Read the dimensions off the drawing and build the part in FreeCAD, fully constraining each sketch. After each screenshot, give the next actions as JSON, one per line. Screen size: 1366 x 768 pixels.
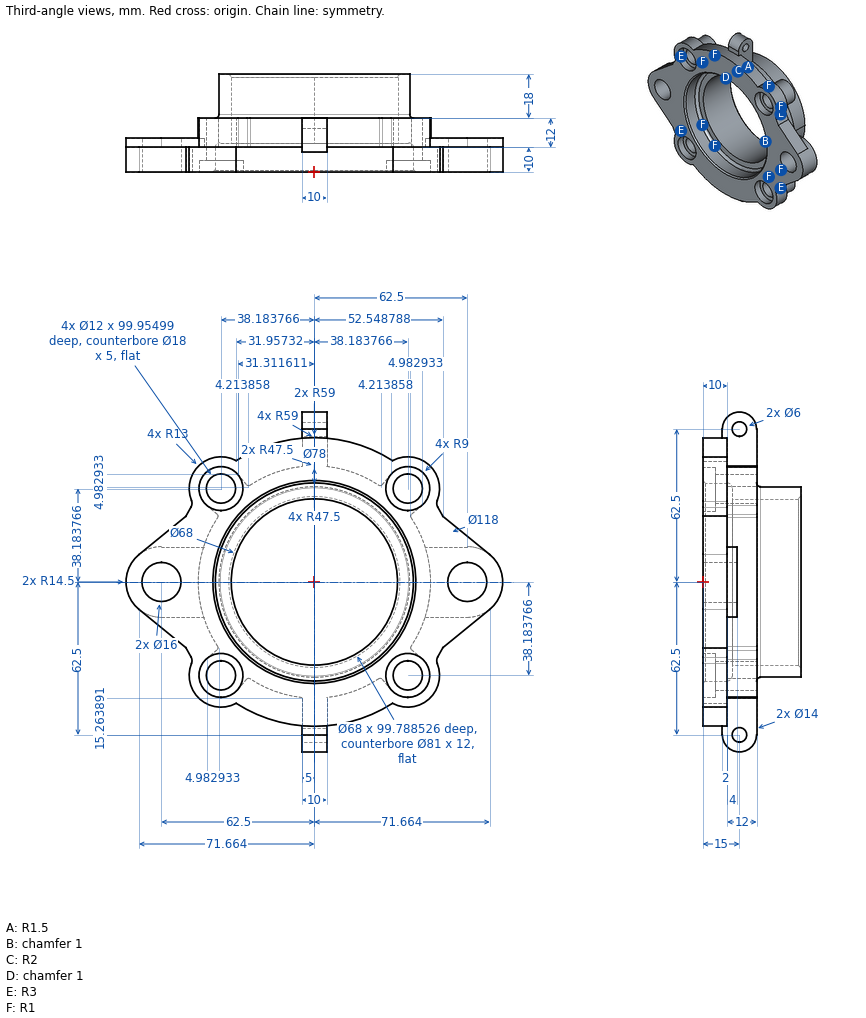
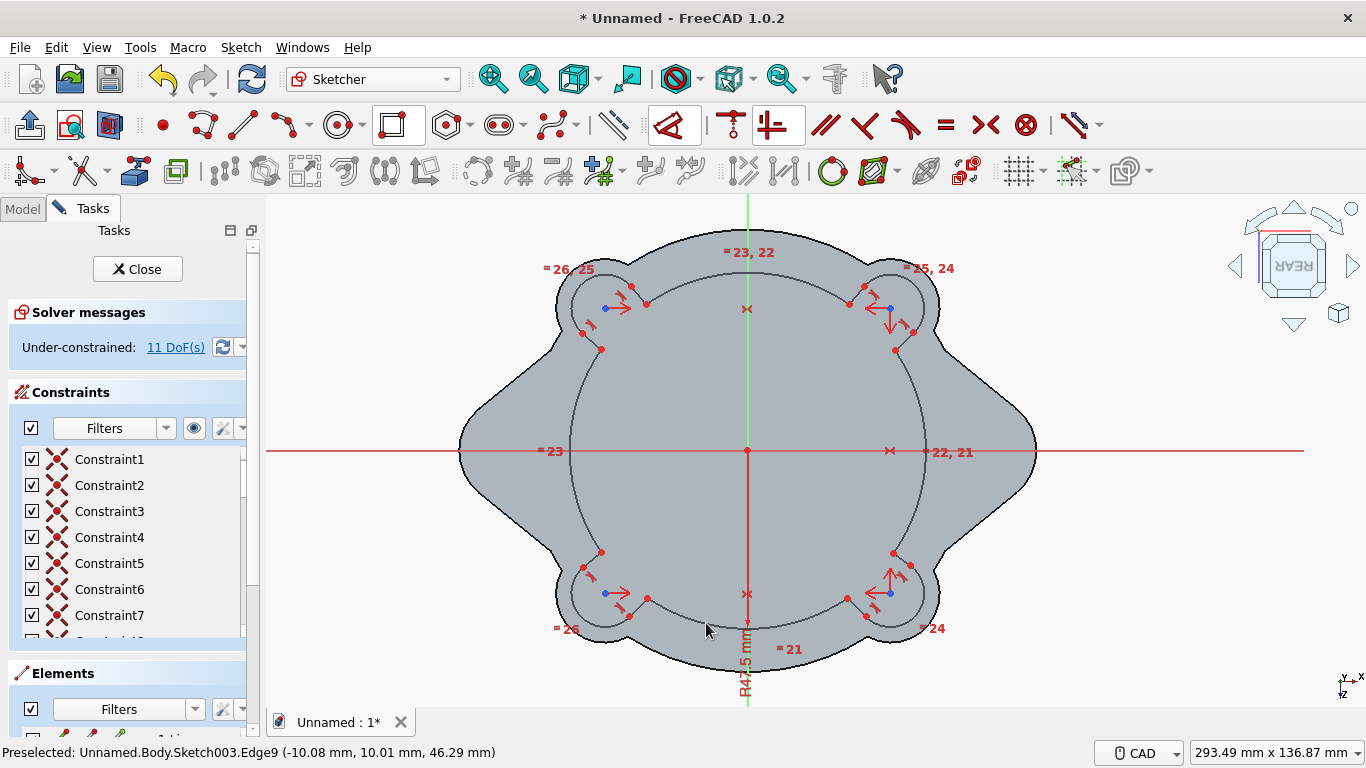
{"action": "left_click", "coordinate": [897, 626]}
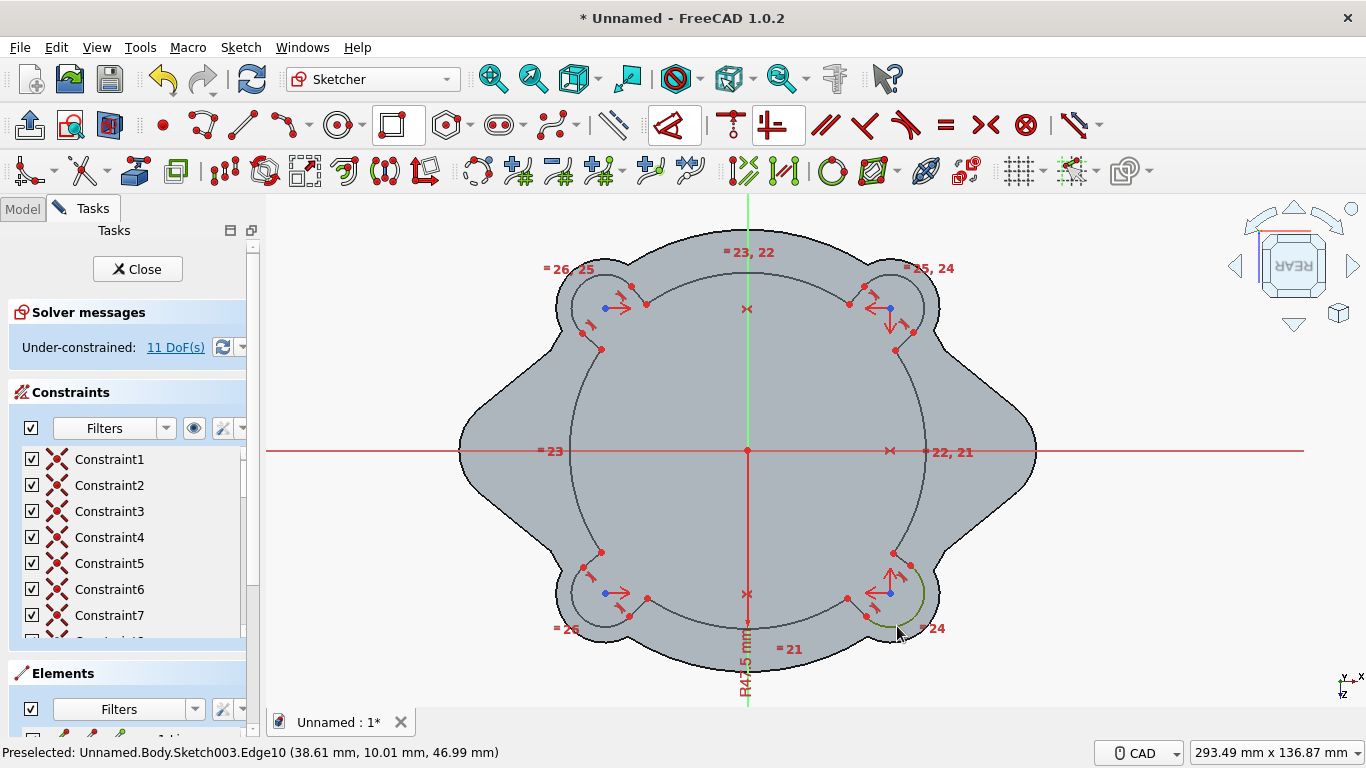
{"action": "key", "text": "k r"}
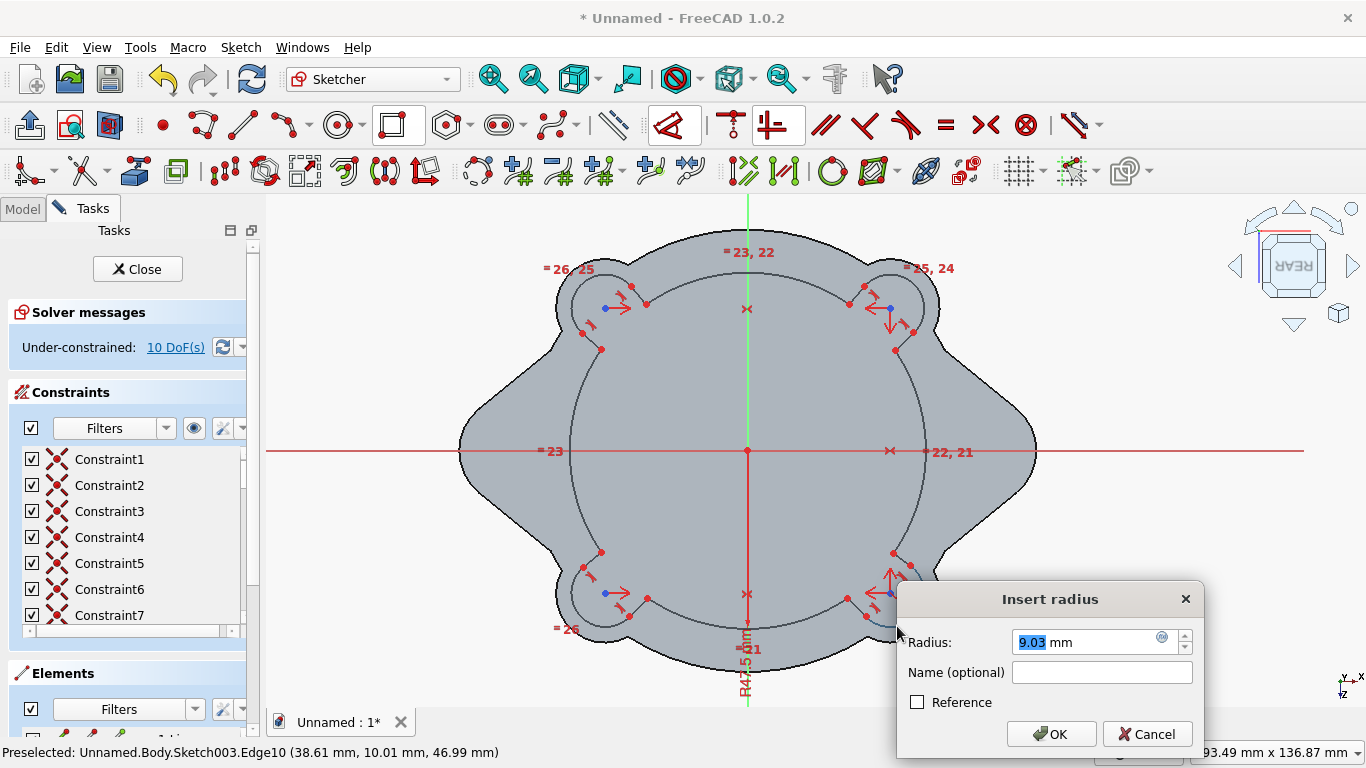
{"action": "type", "text": "9"}
{"action": "key", "text": "Return"}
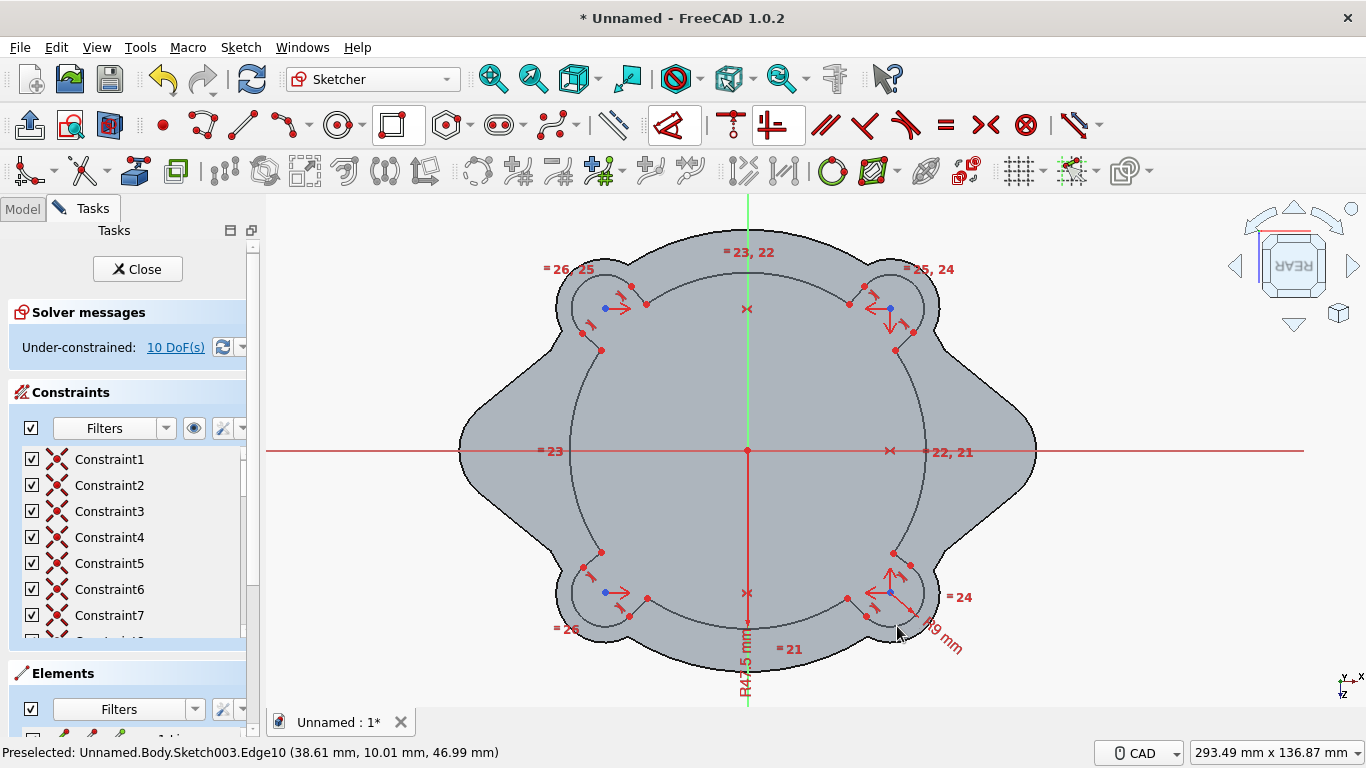
{"action": "scroll", "coordinate": [637, 609], "scroll_direction": "up", "scroll_amount": 5}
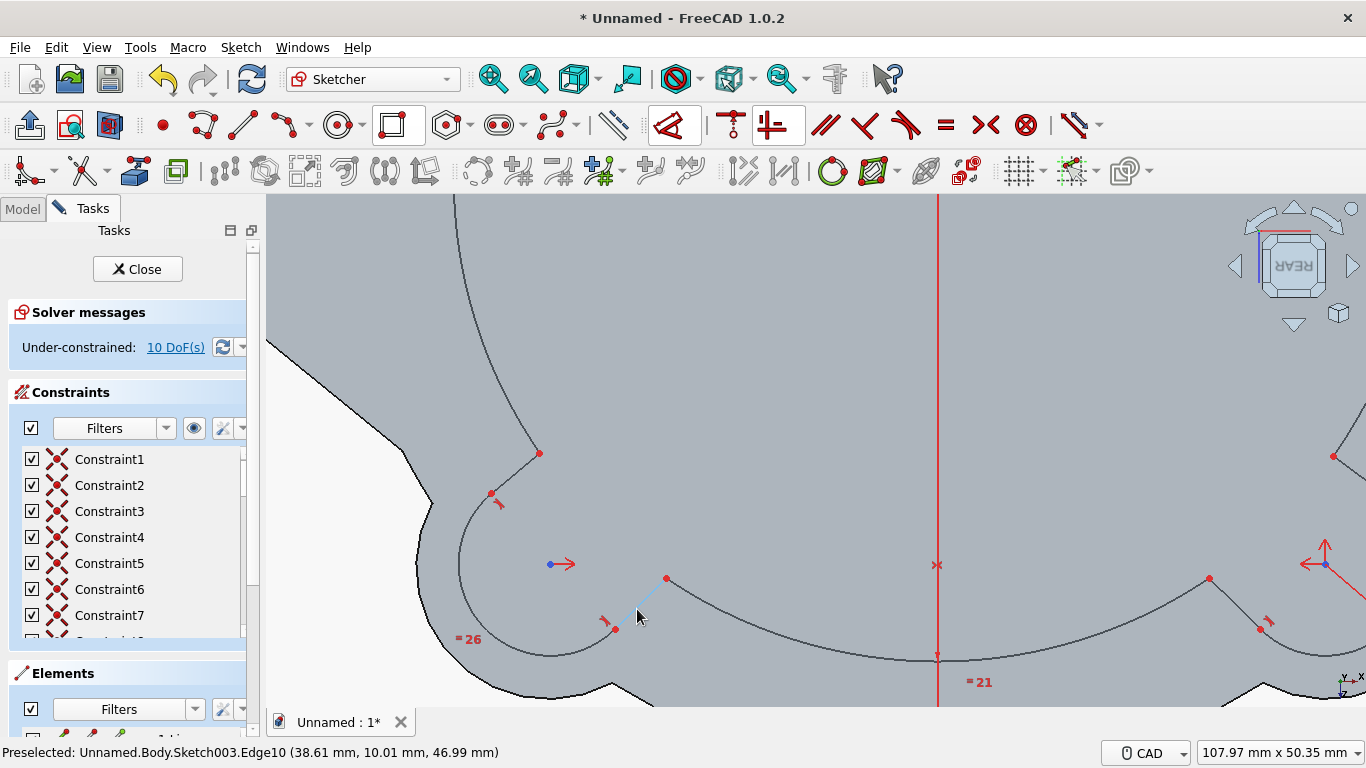
{"action": "left_click", "coordinate": [635, 609]}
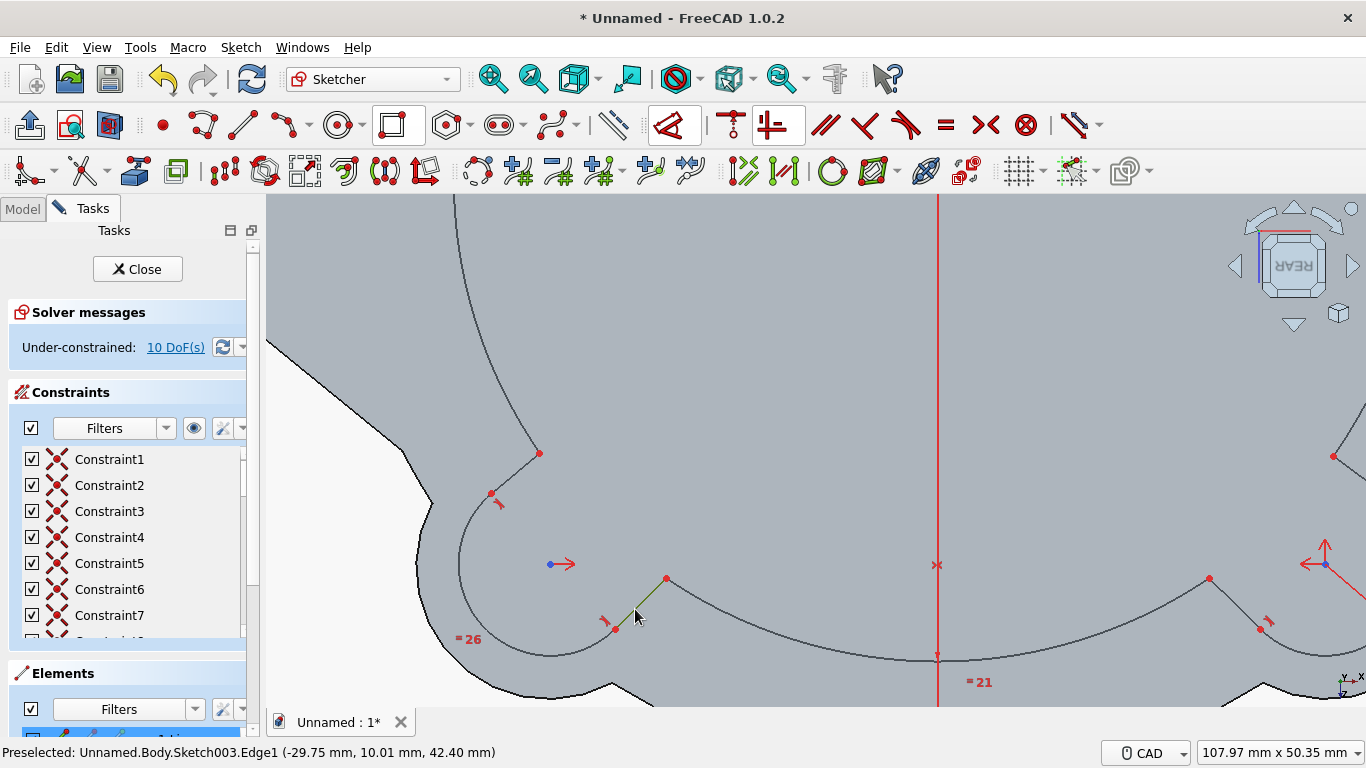
{"action": "left_click", "coordinate": [696, 126]}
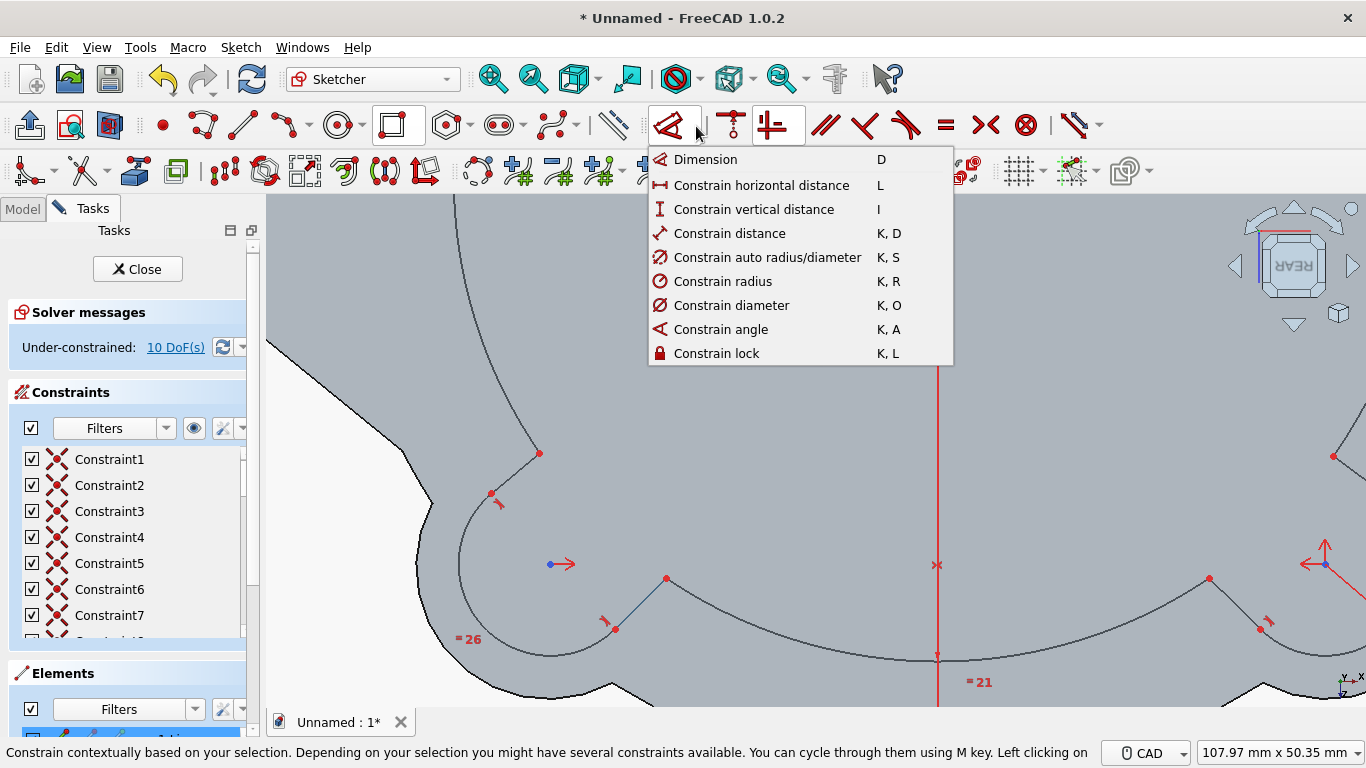
{"action": "left_click", "coordinate": [801, 185]}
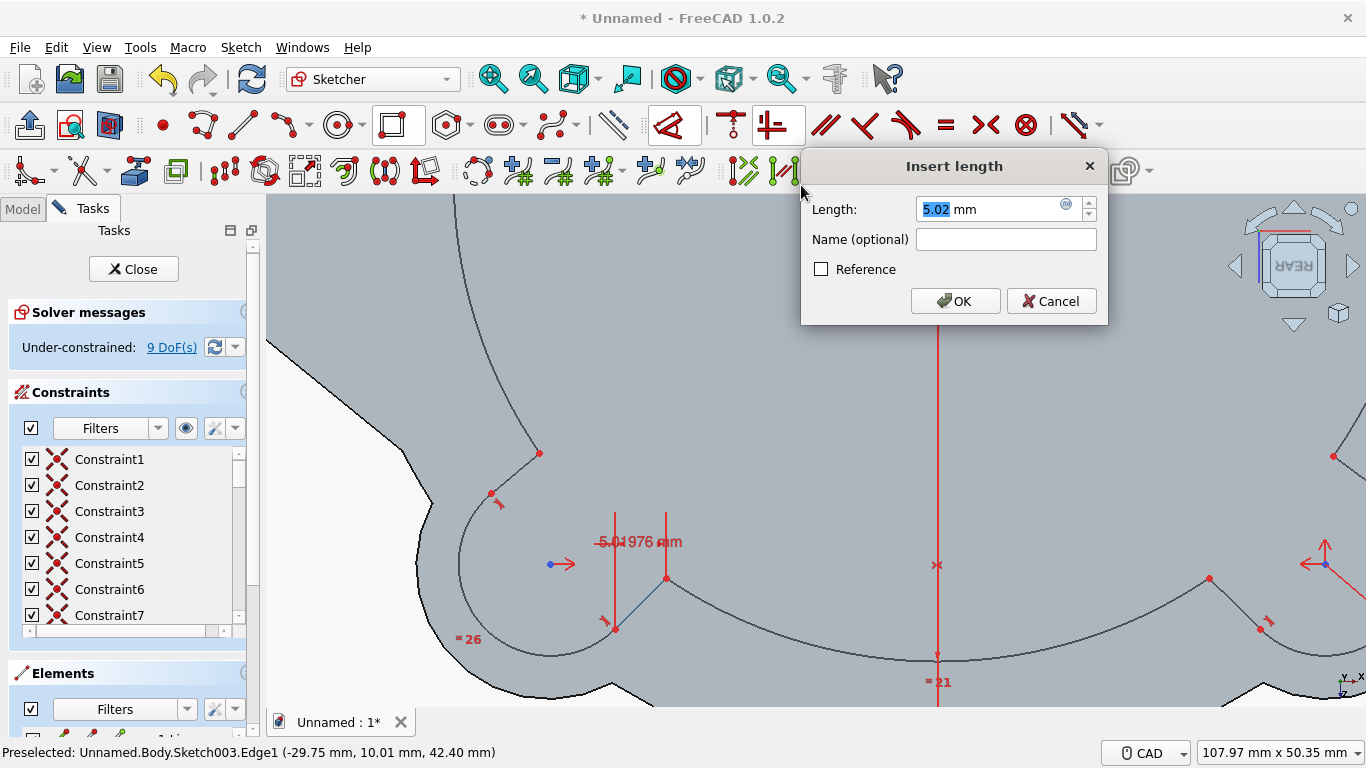
{"action": "type", "text": "4.213858"}
{"action": "key", "text": "Return"}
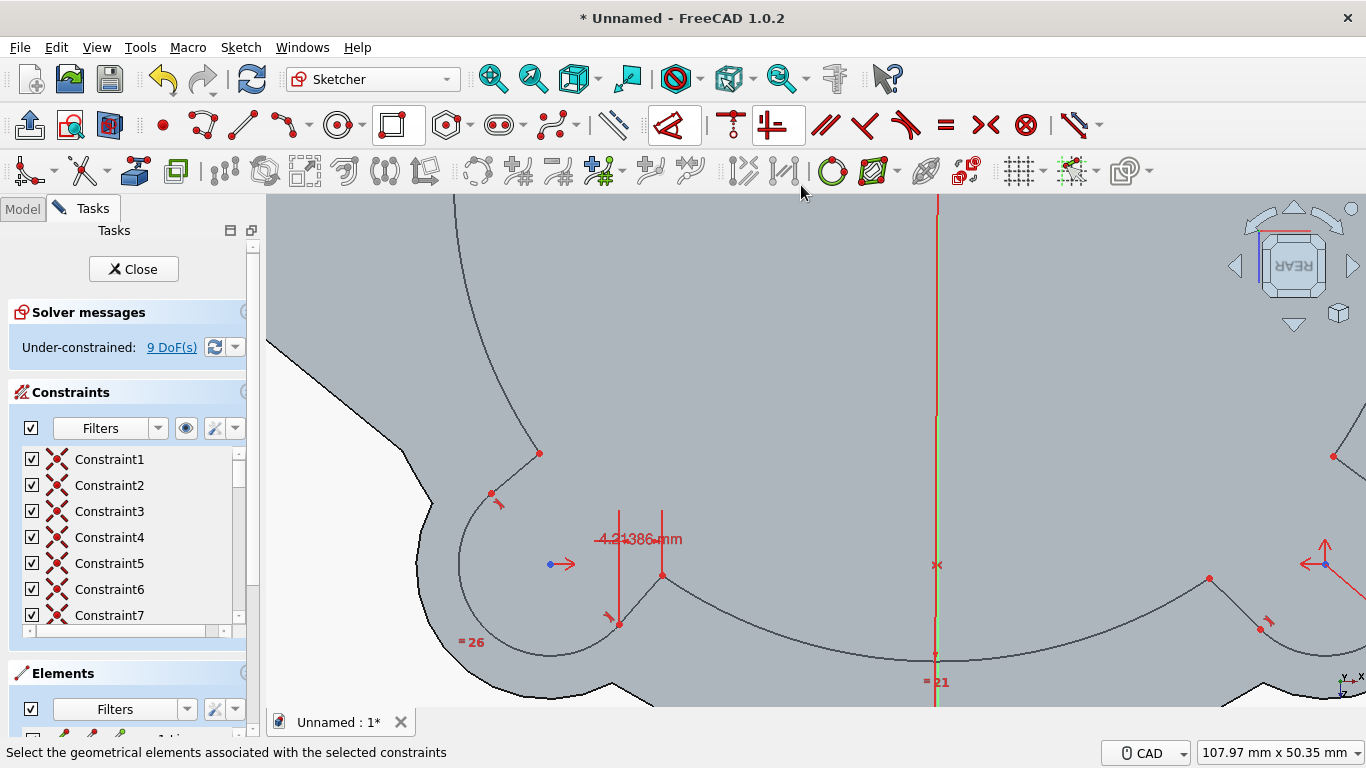
{"action": "left_click", "coordinate": [632, 610]}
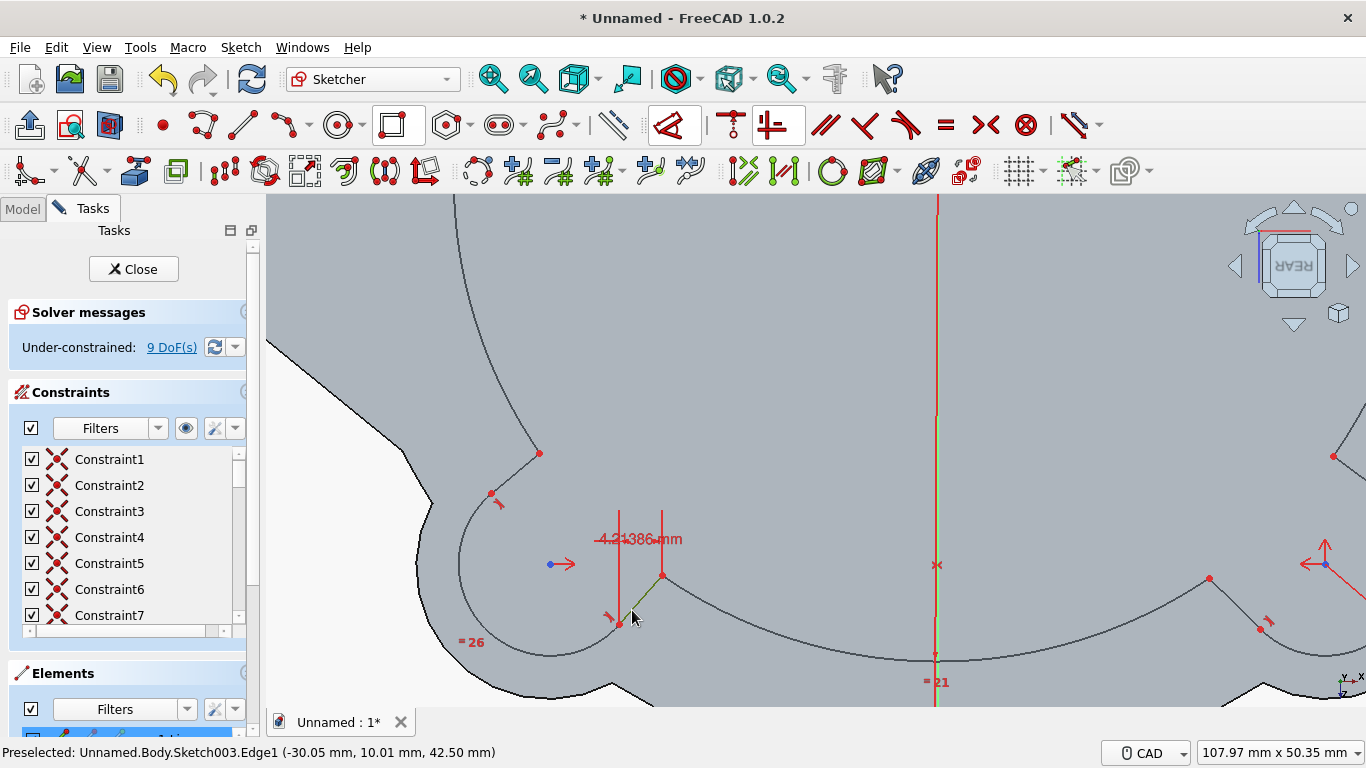
{"action": "key", "text": "i"}